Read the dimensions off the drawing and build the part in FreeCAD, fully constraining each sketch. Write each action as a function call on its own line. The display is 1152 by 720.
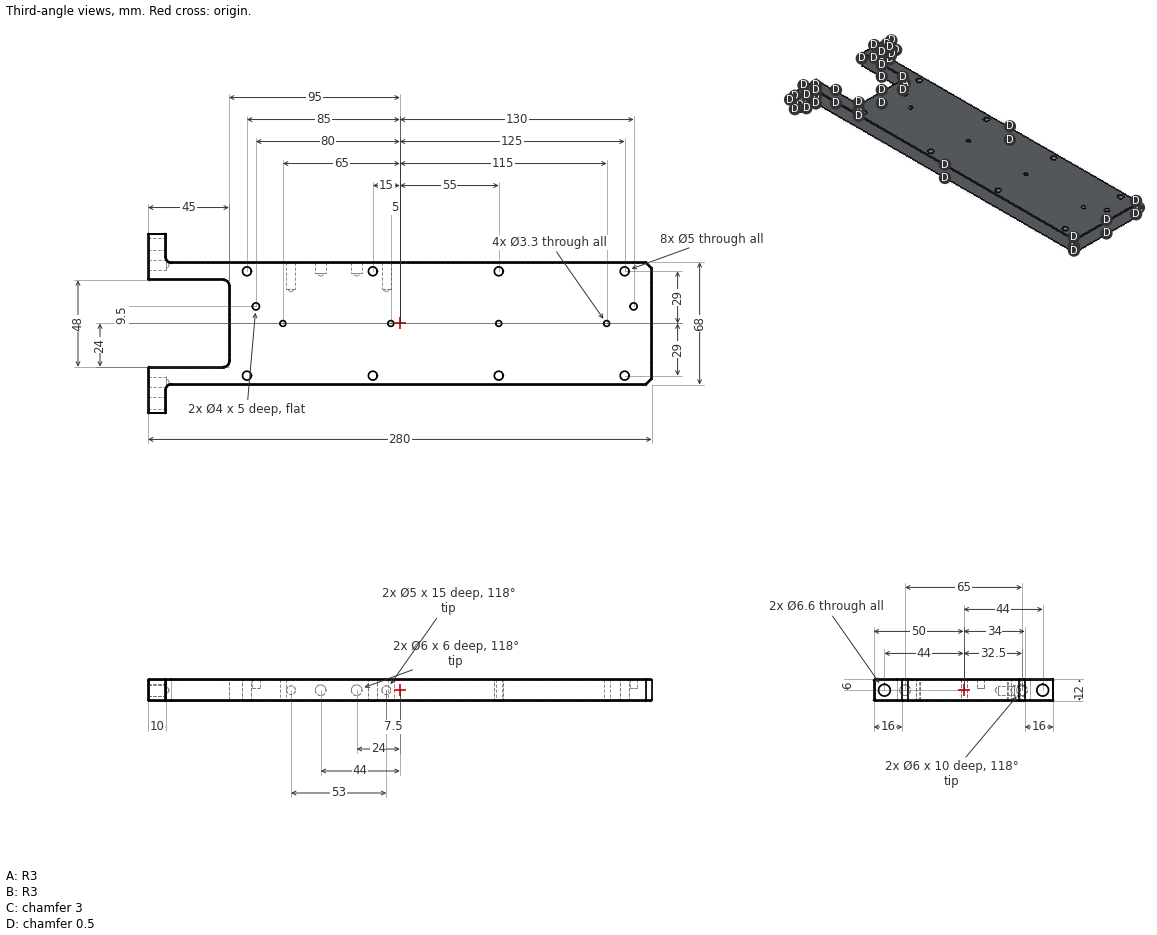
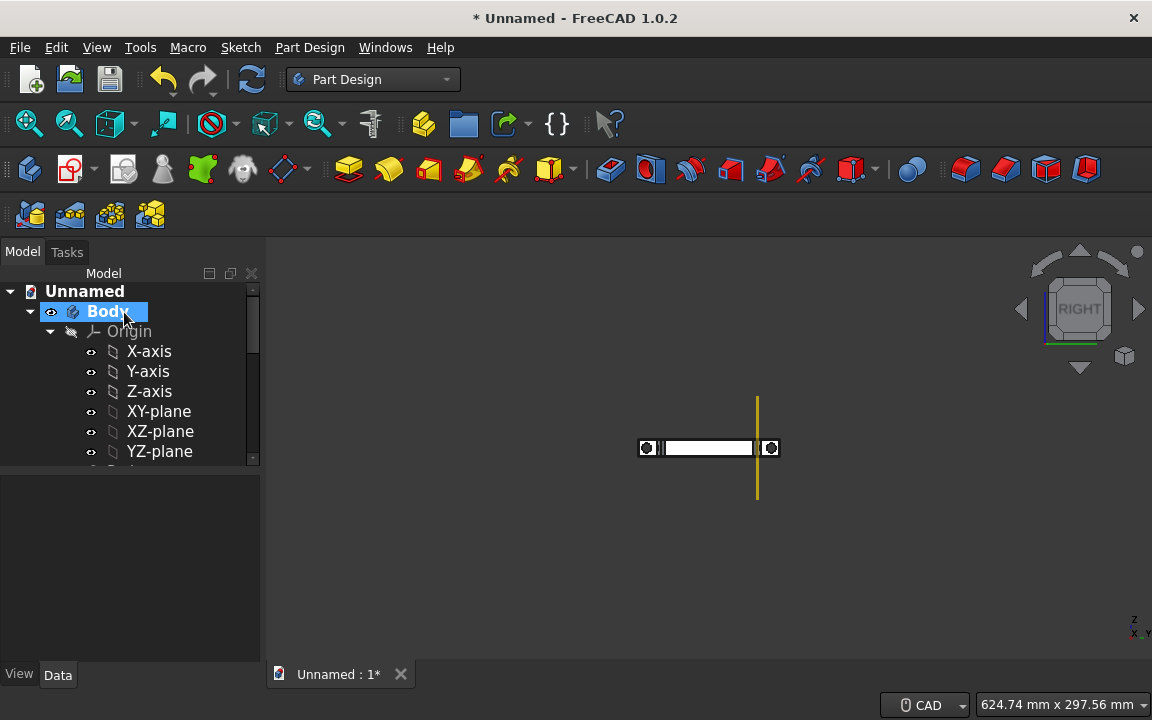
scroll(100, 367, down, 3)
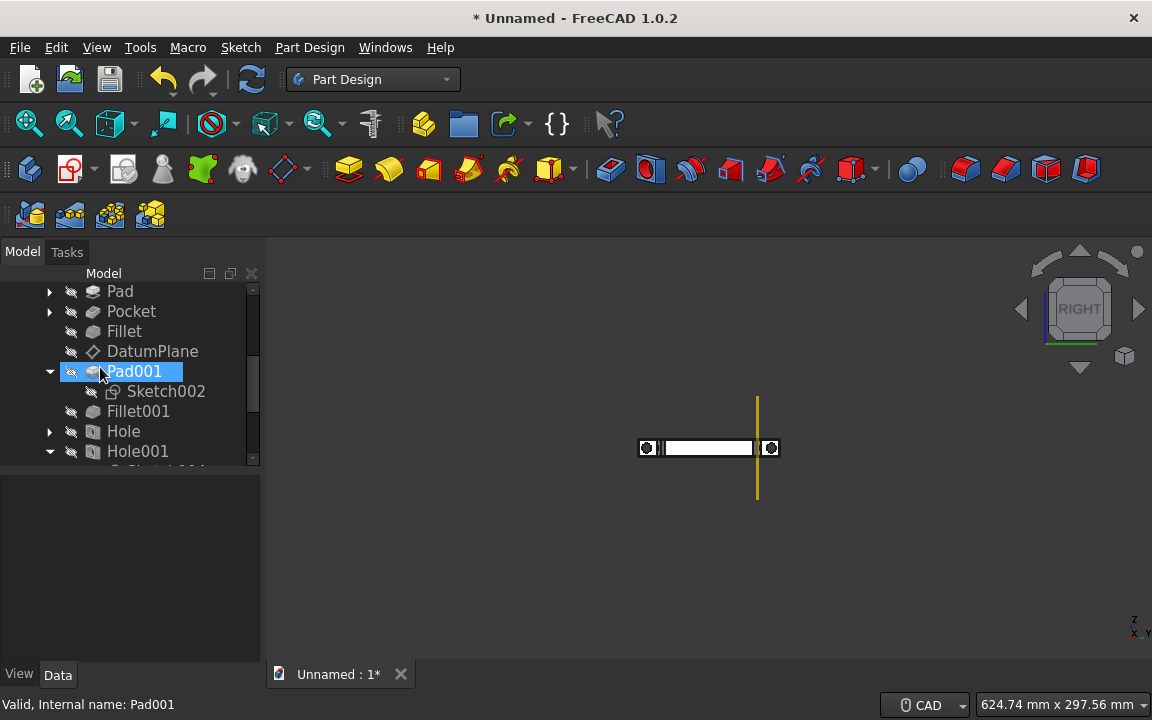
scroll(140, 367, up, 15)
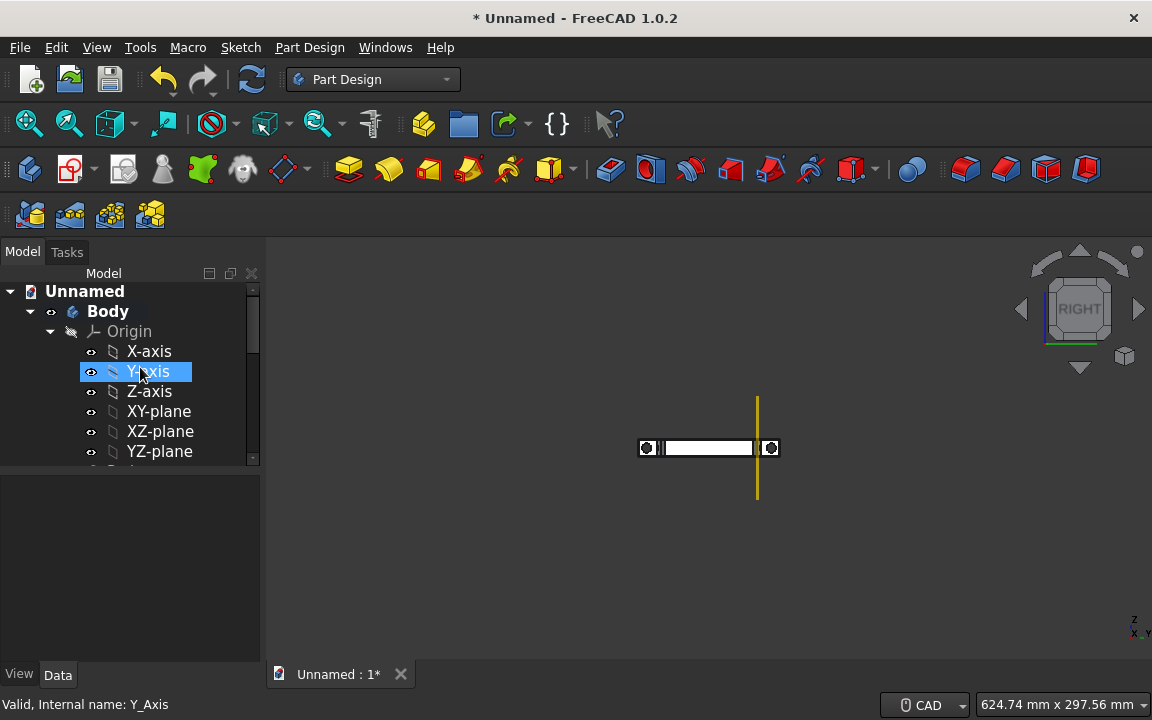
scroll(100, 367, down, 6)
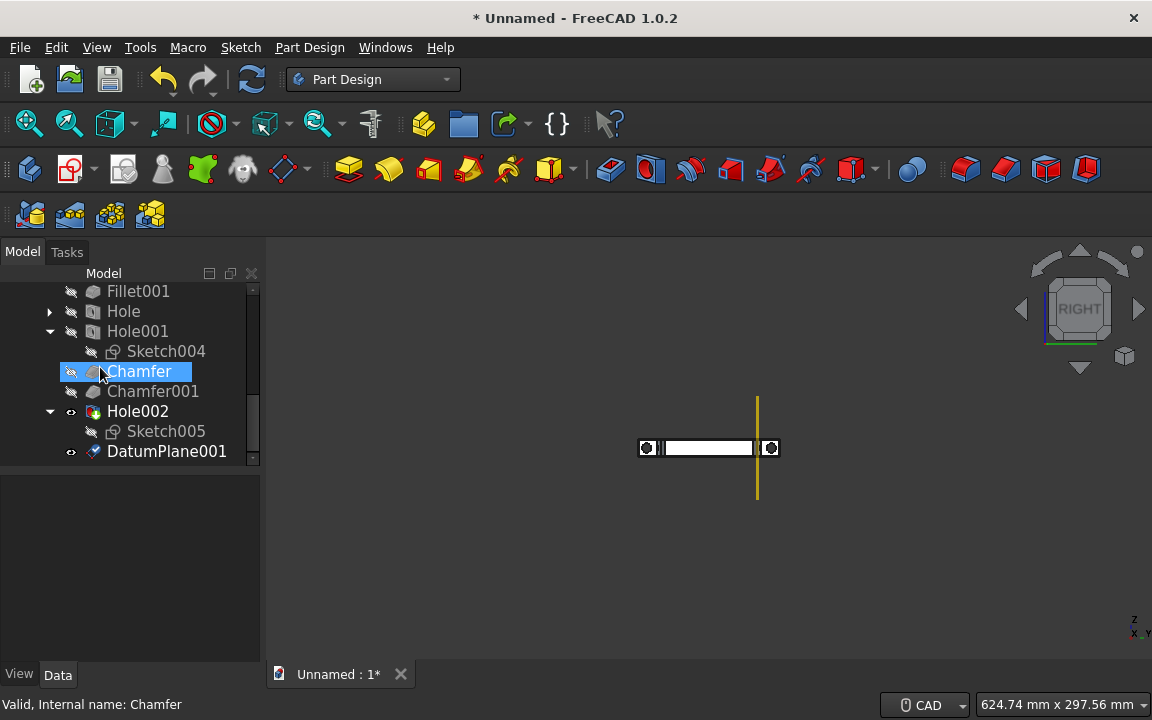
click(116, 452)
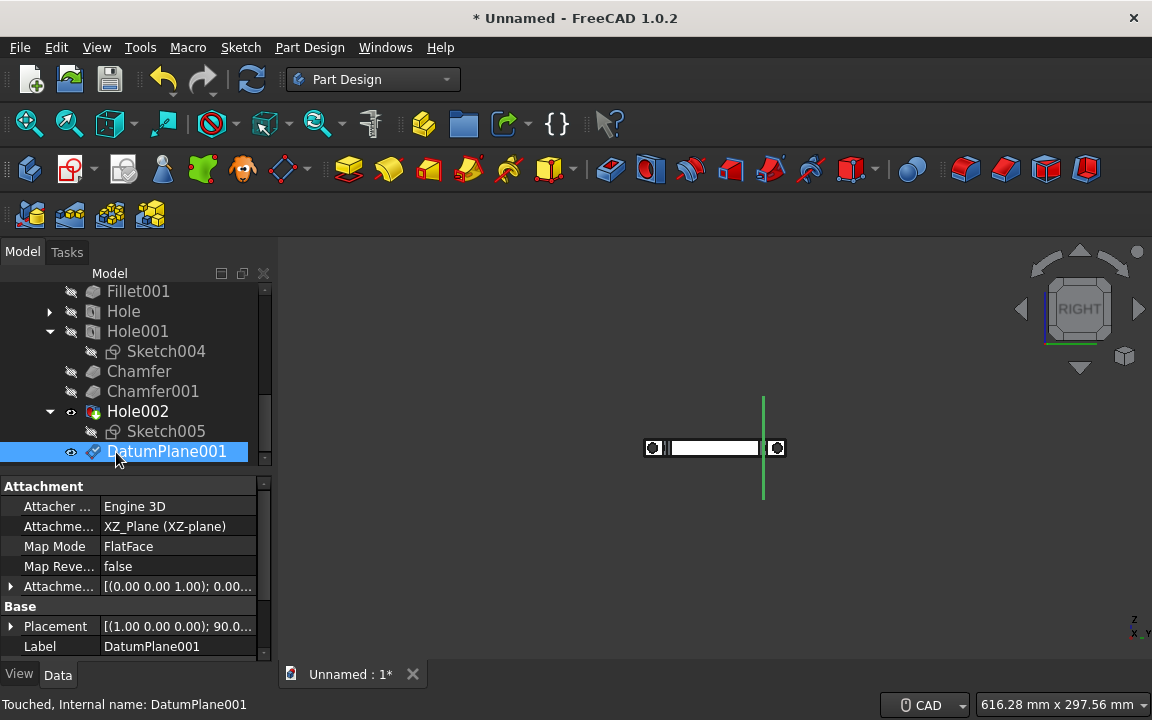
click(70, 170)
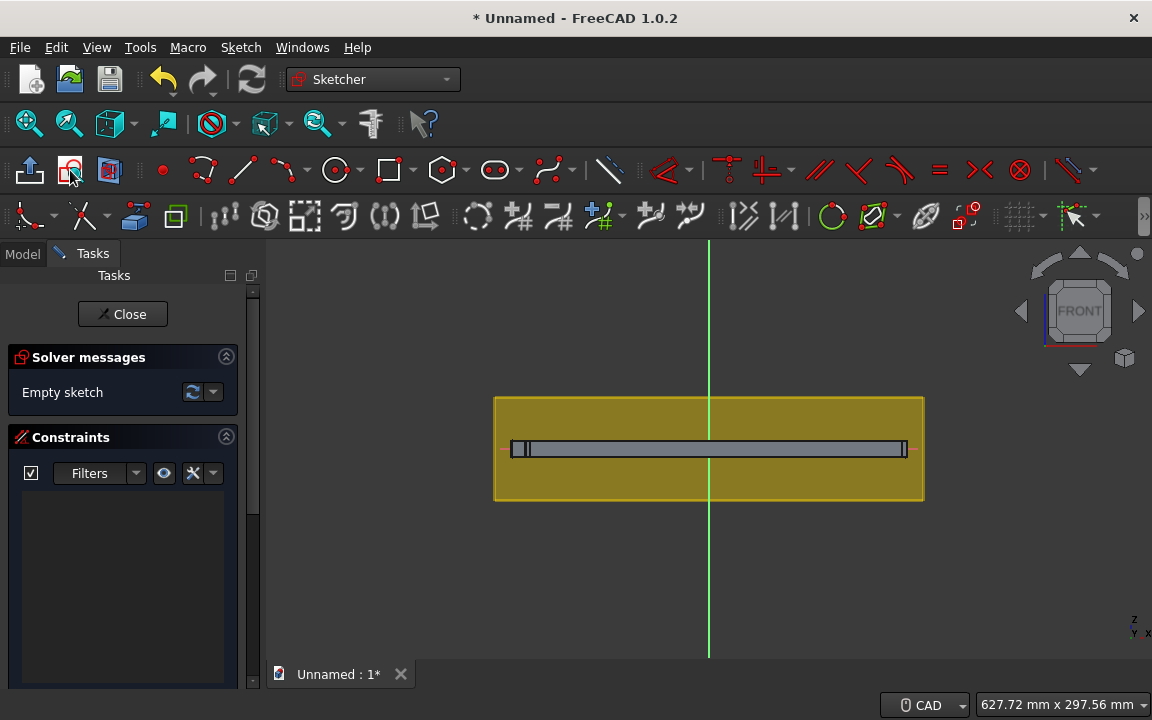
key(q)
key(s)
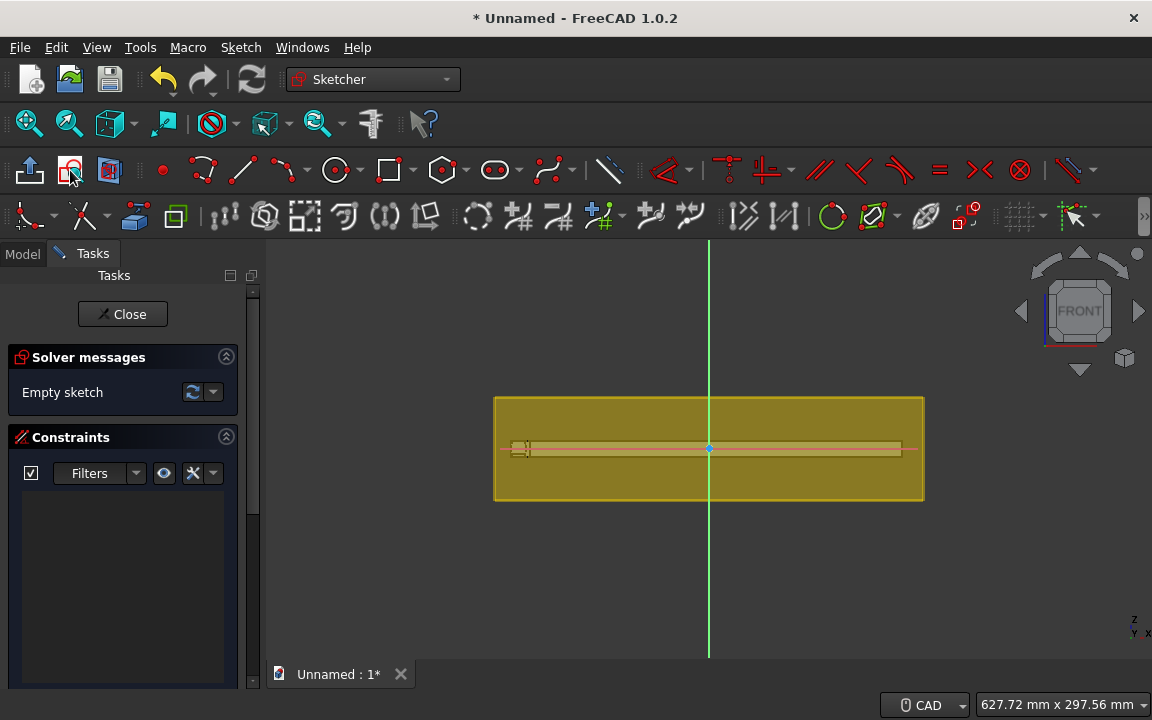
scroll(681, 449, up, 10)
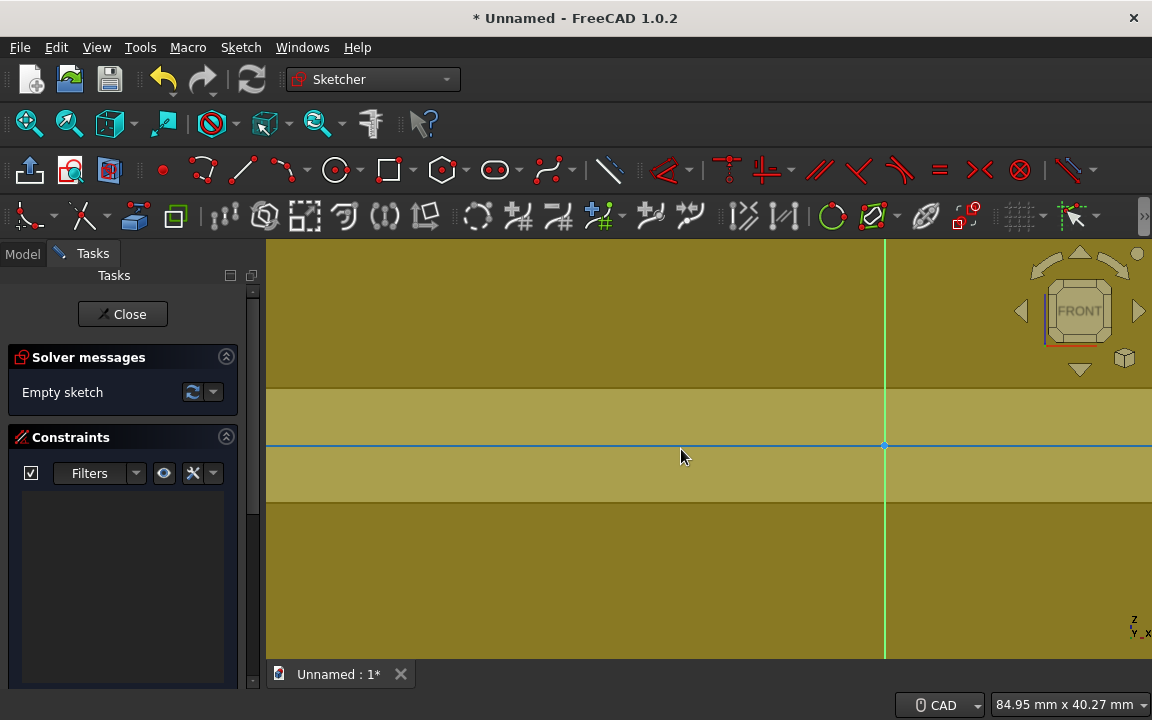
key(g)
key(c)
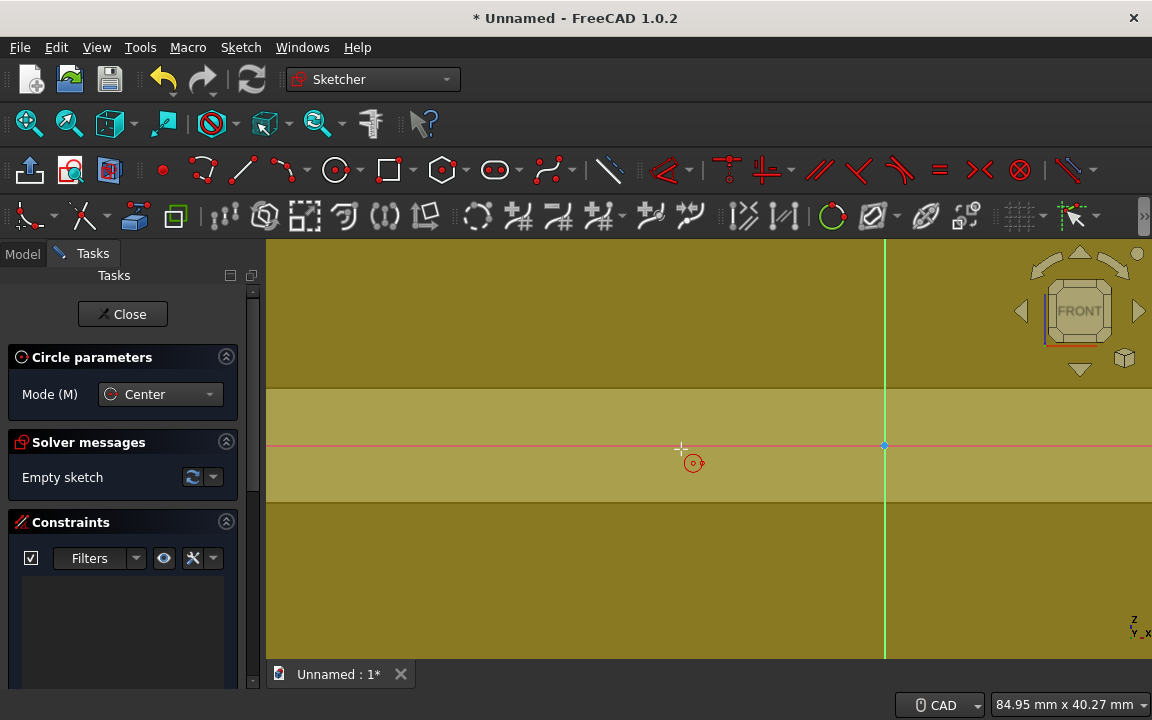
click(635, 446)
move(657, 424)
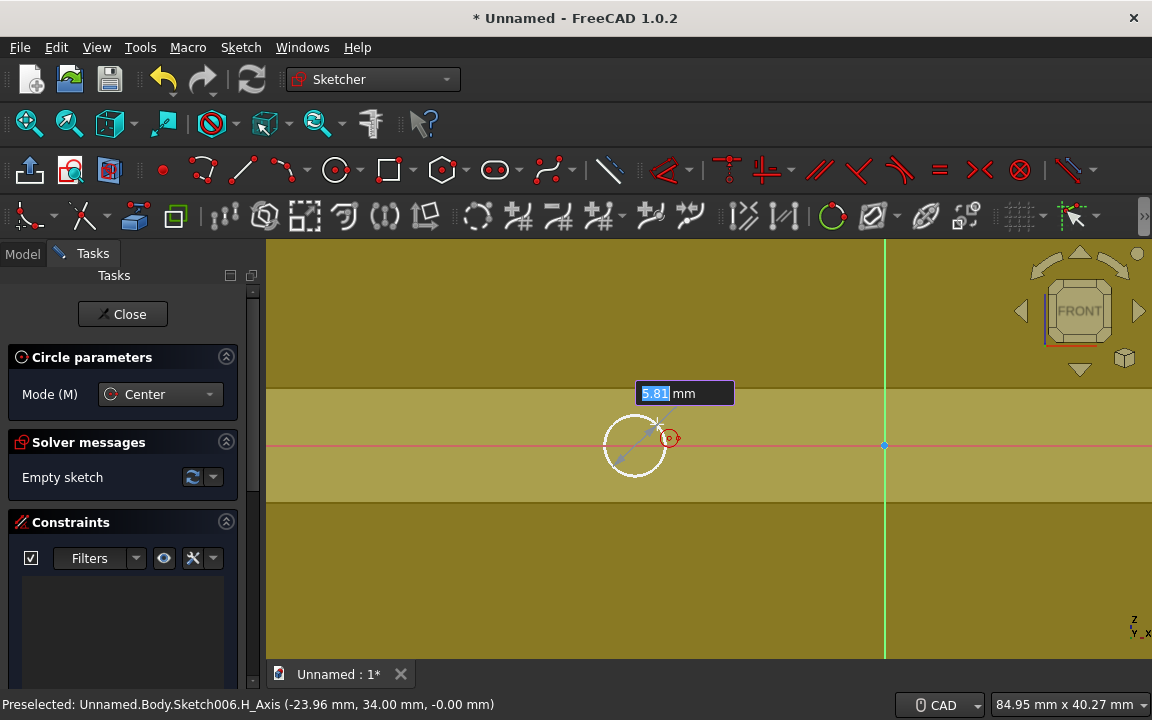
text(6)
key(Return)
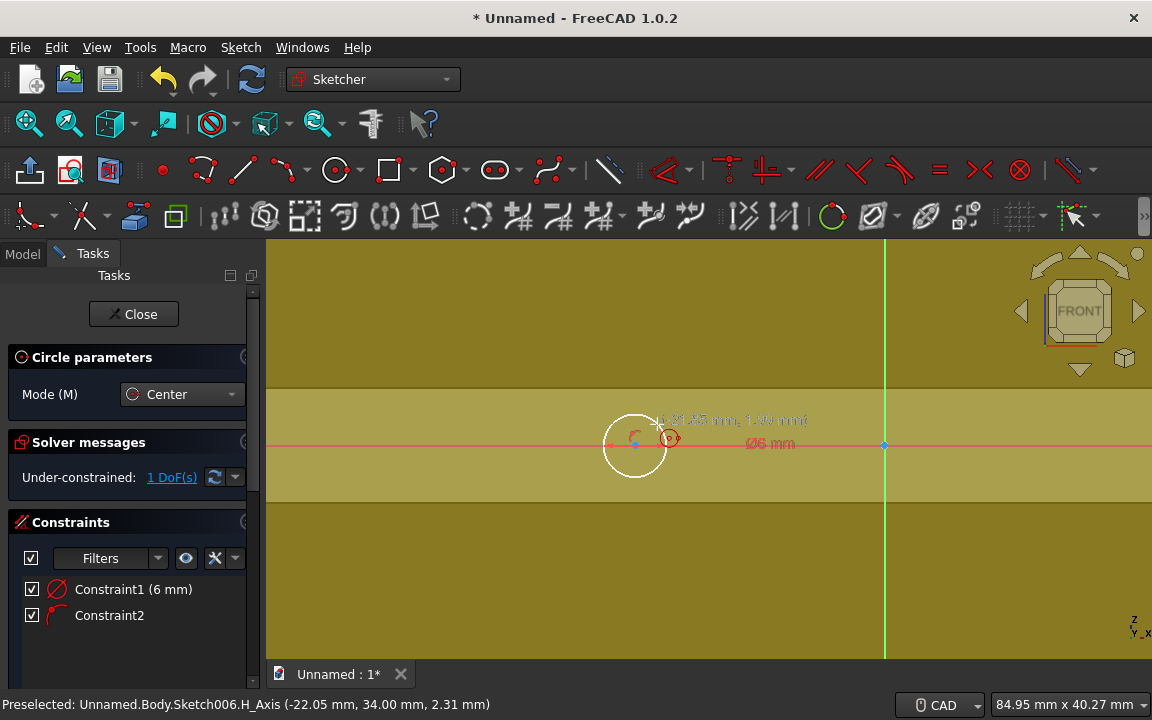
click(426, 446)
move(448, 424)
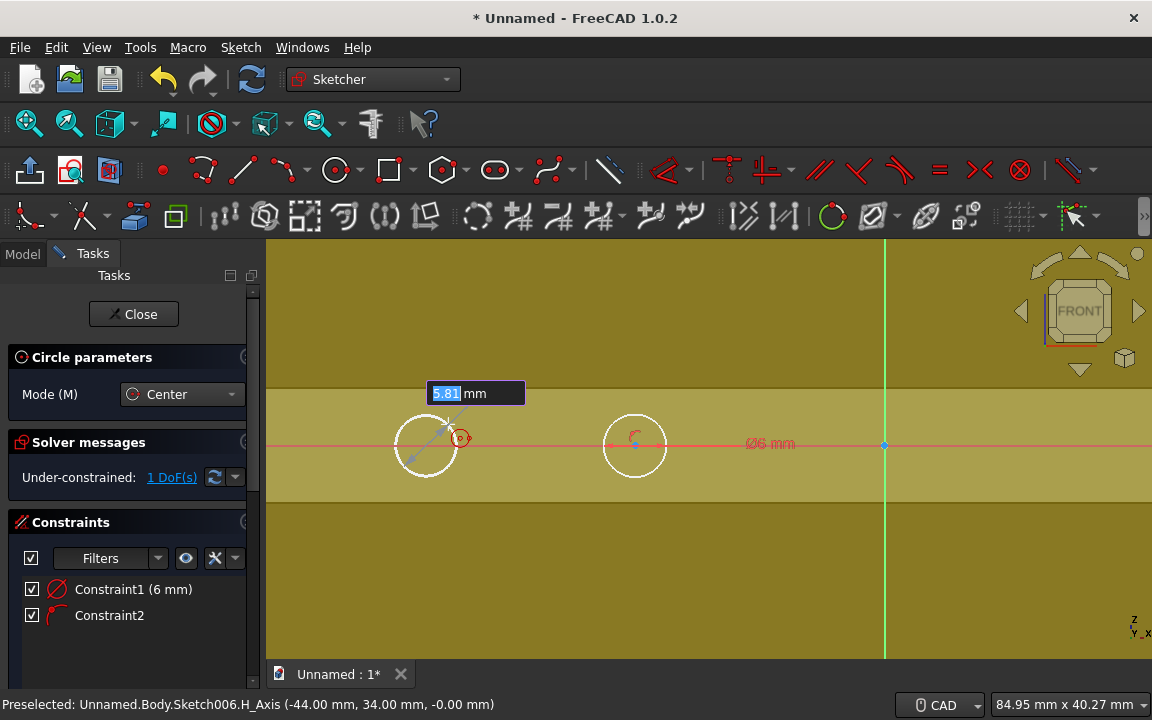
text(6)
key(Return)
key(Escape)